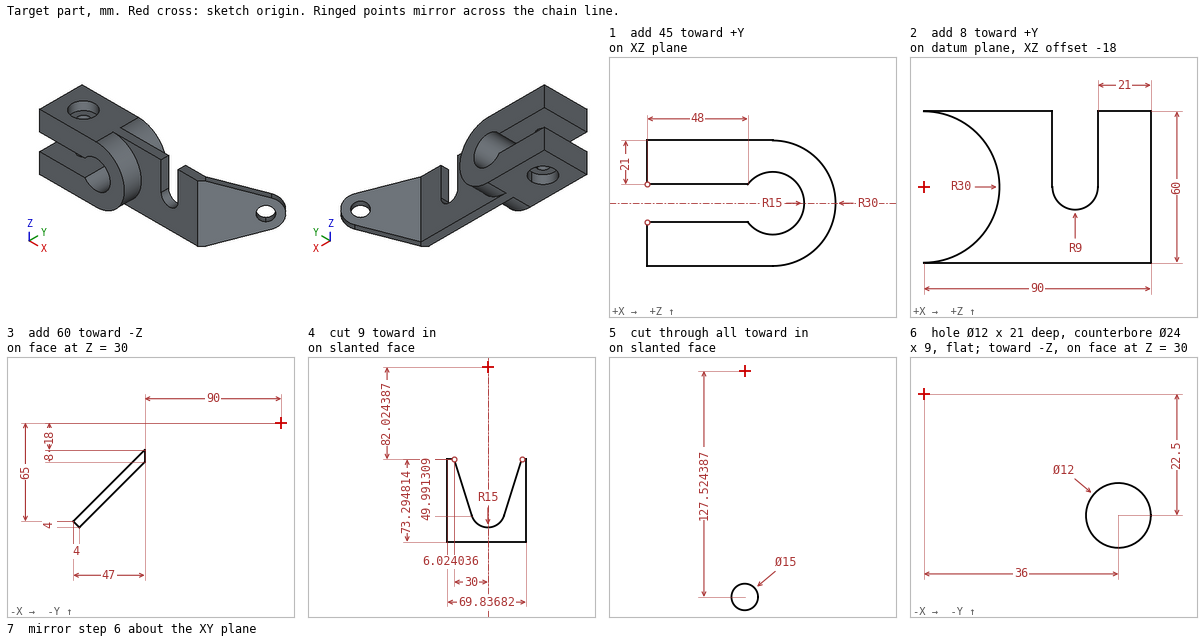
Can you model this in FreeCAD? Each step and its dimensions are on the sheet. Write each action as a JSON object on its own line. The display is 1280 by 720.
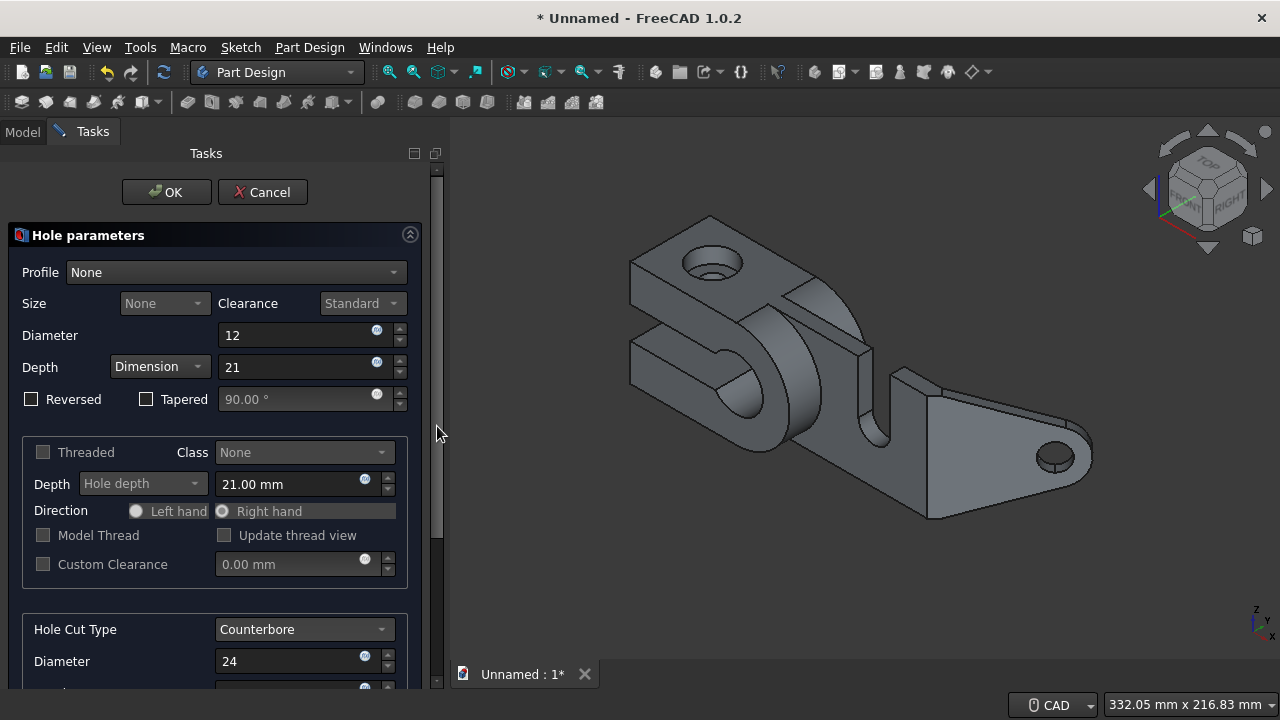
{"action": "left_click", "coordinate": [167, 192]}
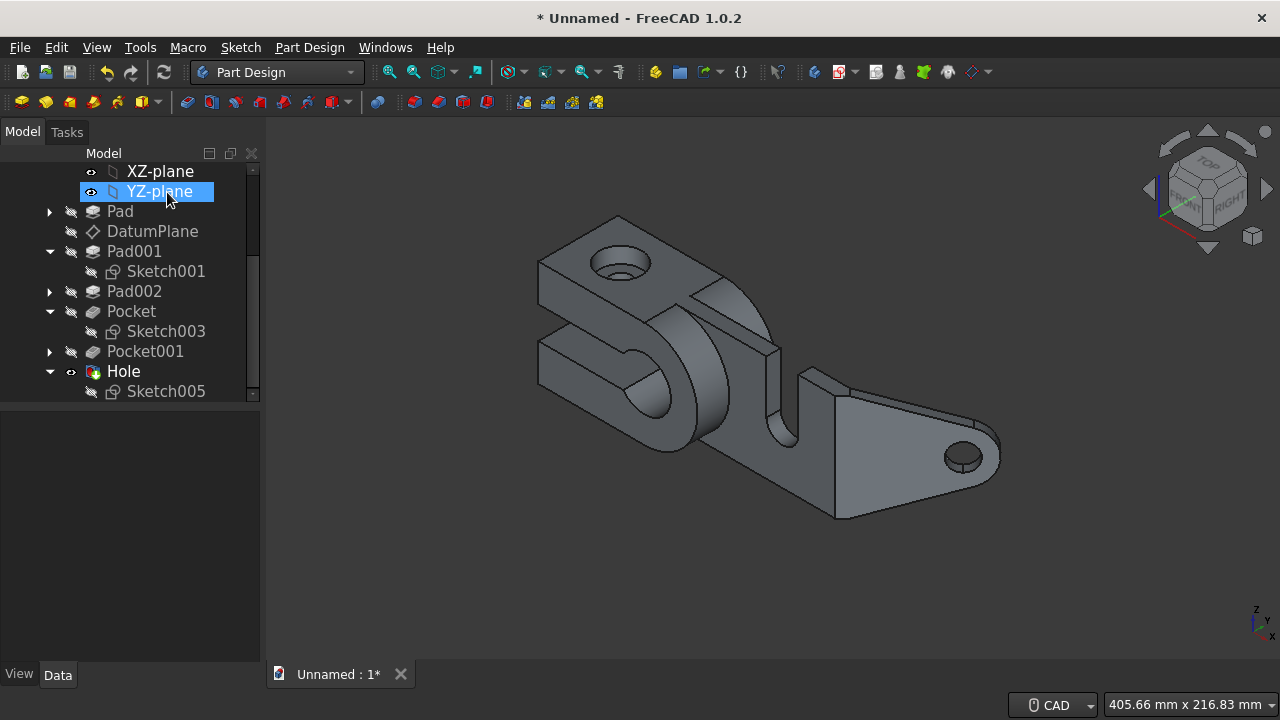
{"action": "left_click", "coordinate": [116, 372]}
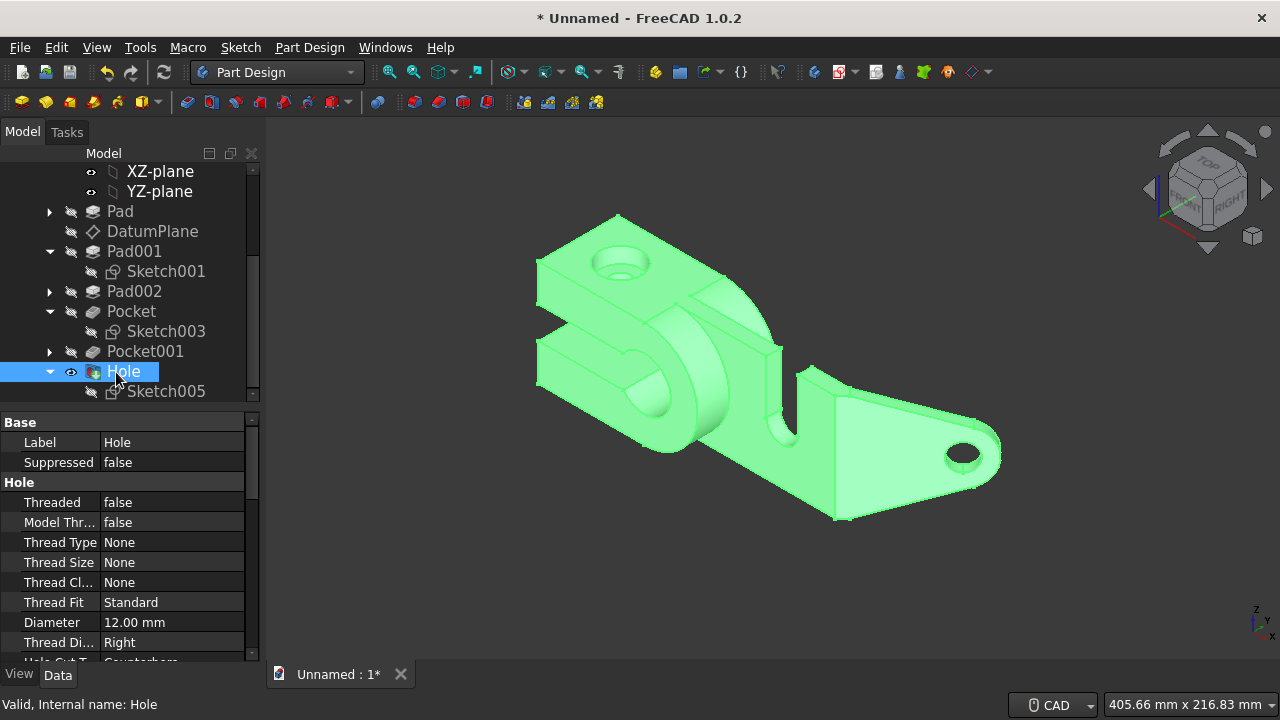
{"action": "left_click", "coordinate": [524, 102]}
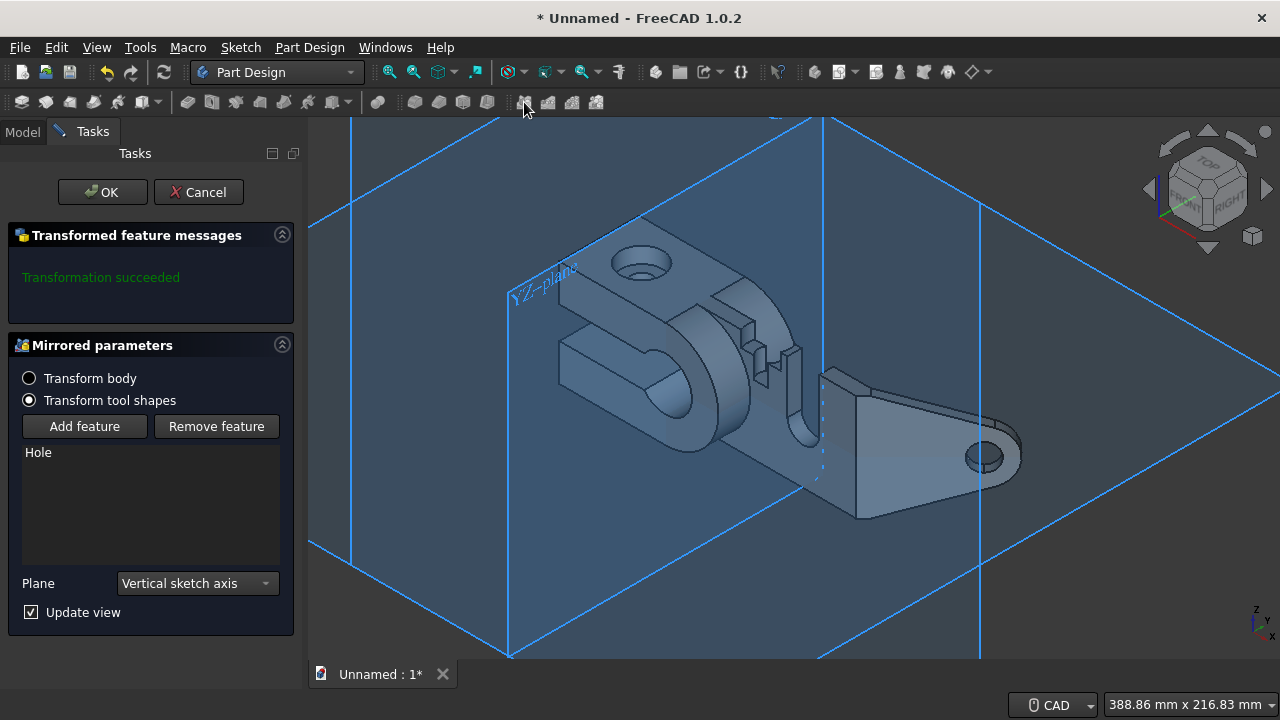
{"action": "left_click", "coordinate": [198, 584]}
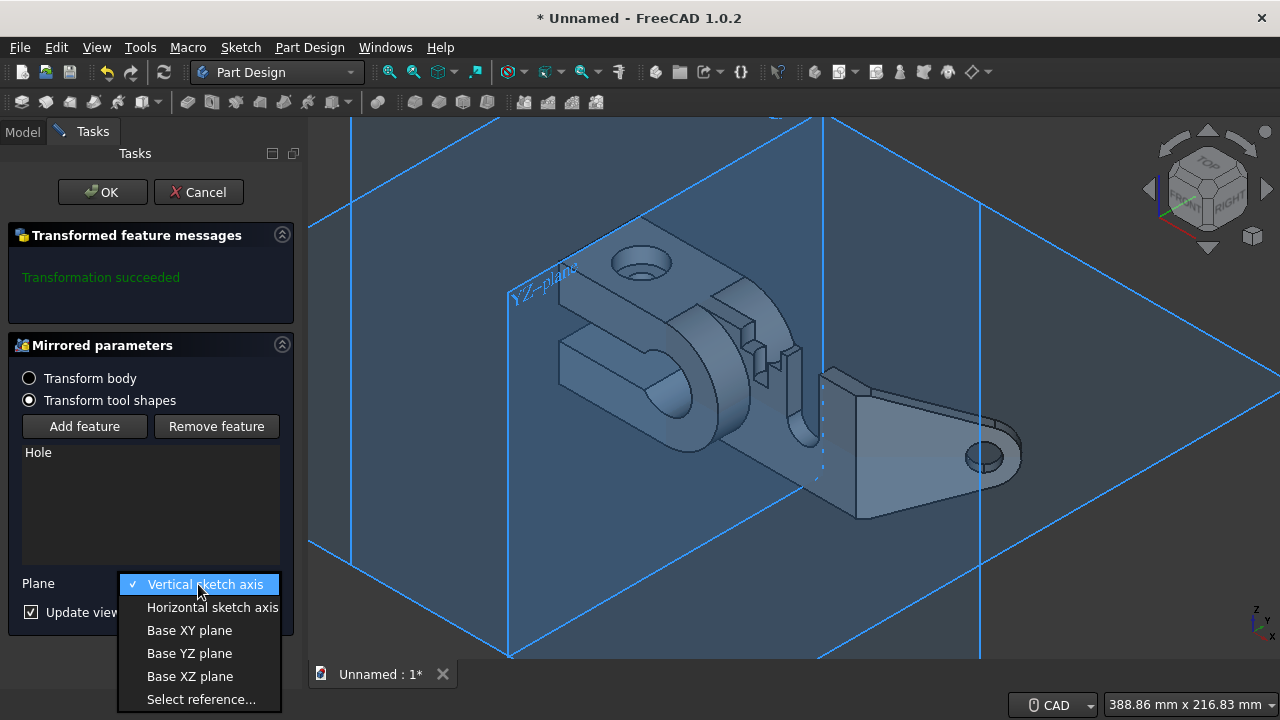
{"action": "left_click", "coordinate": [198, 630]}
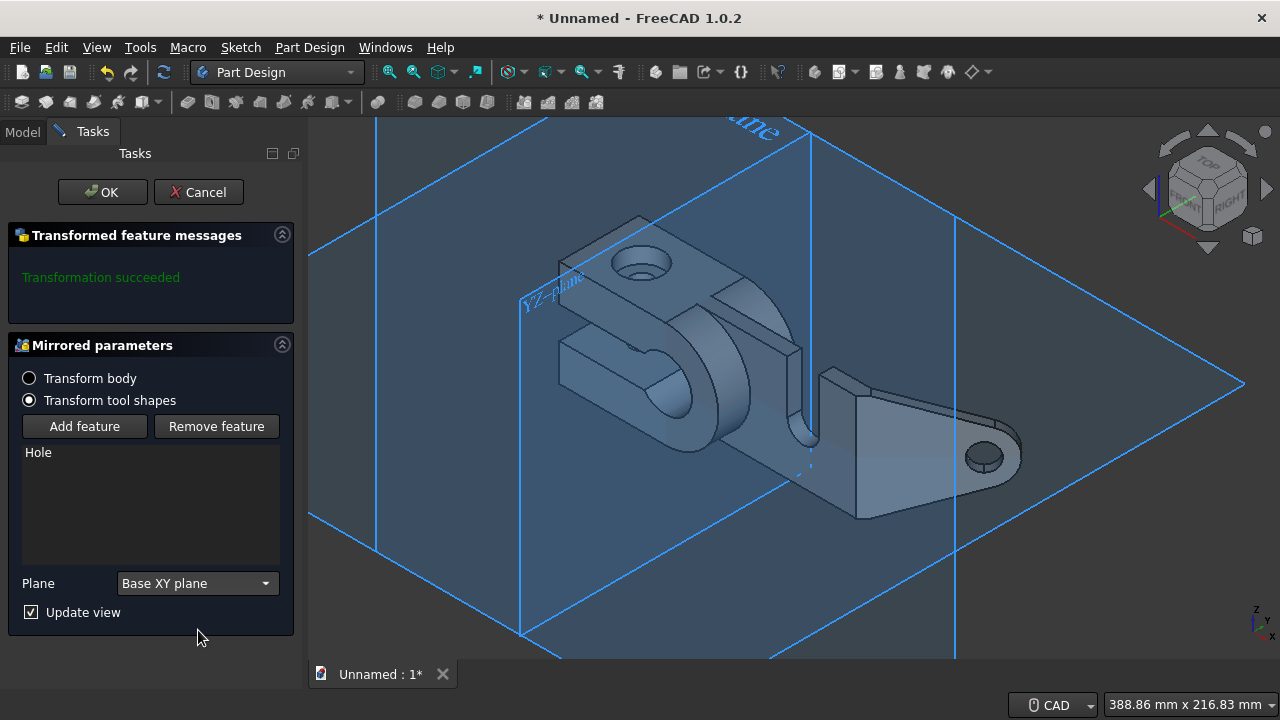
{"action": "left_click", "coordinate": [103, 192]}